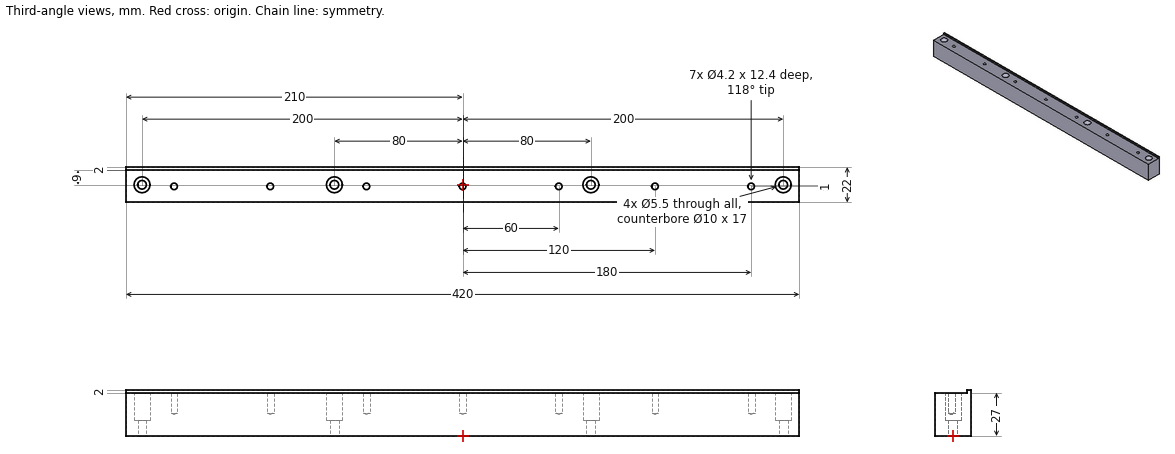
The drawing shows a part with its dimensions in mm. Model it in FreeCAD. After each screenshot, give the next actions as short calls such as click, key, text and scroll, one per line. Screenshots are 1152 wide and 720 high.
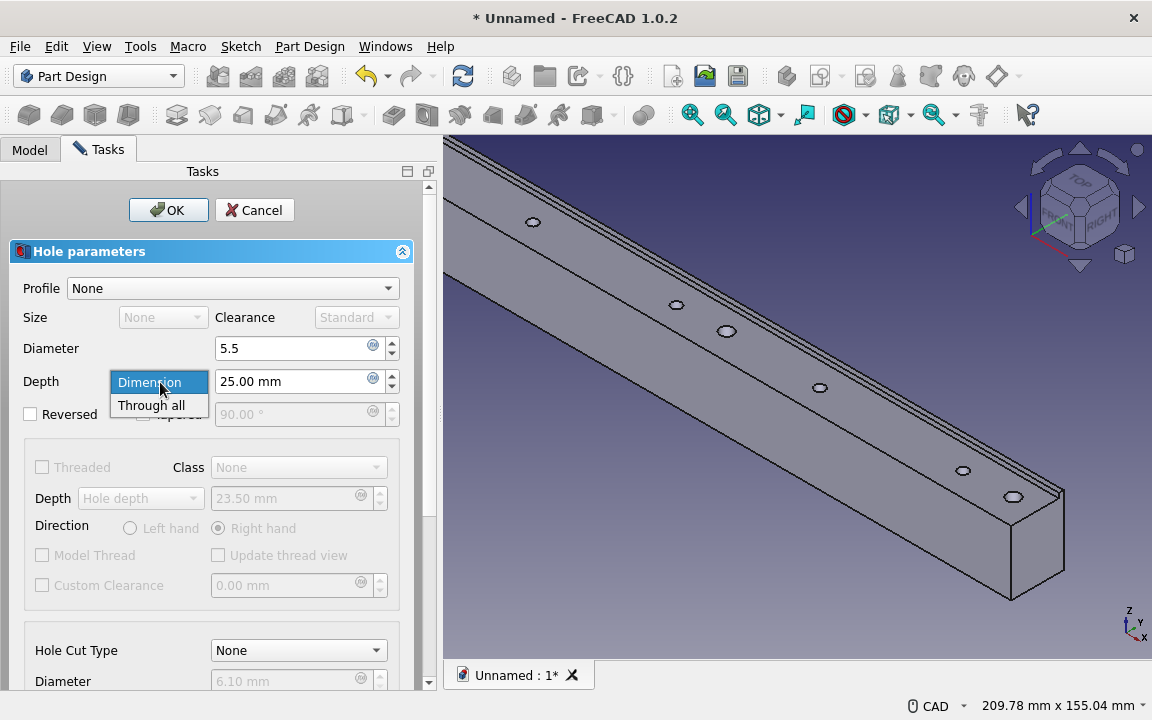
click(158, 406)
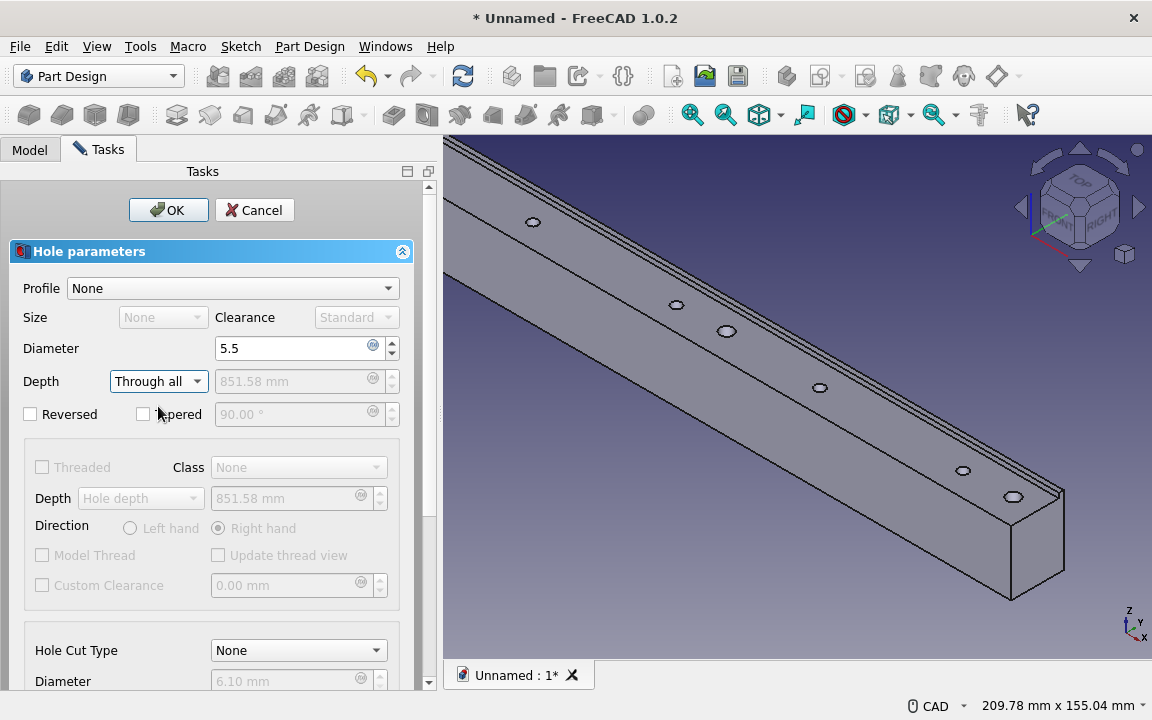
click(300, 650)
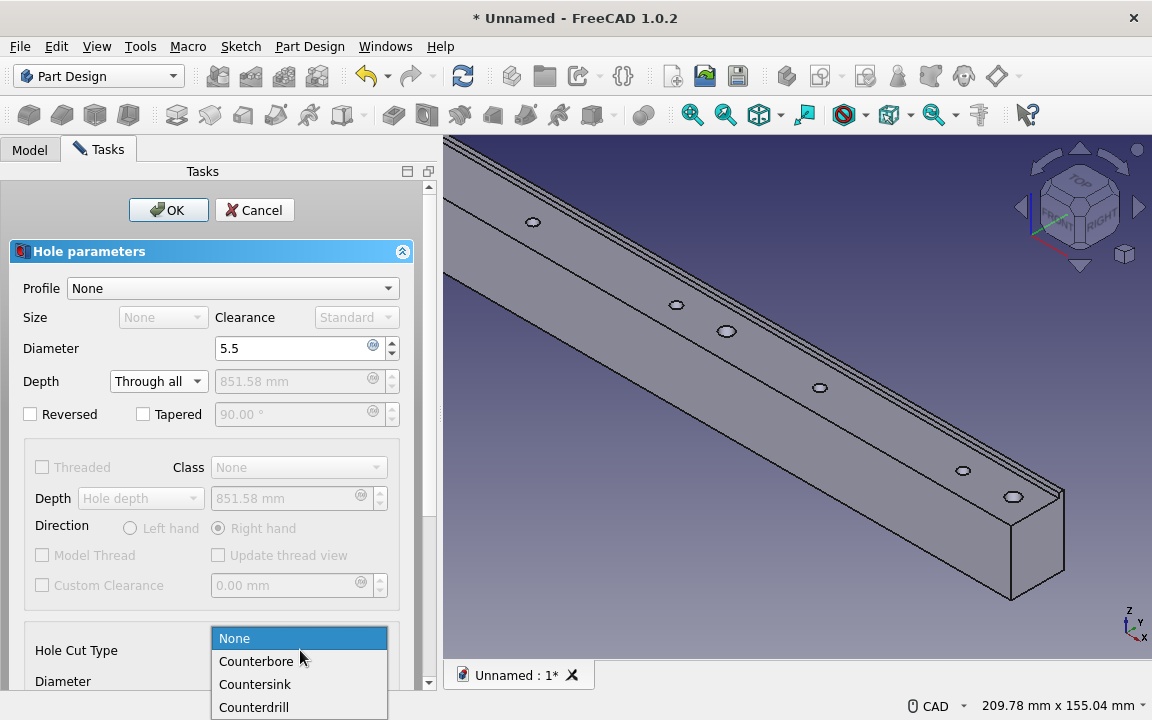
click(298, 662)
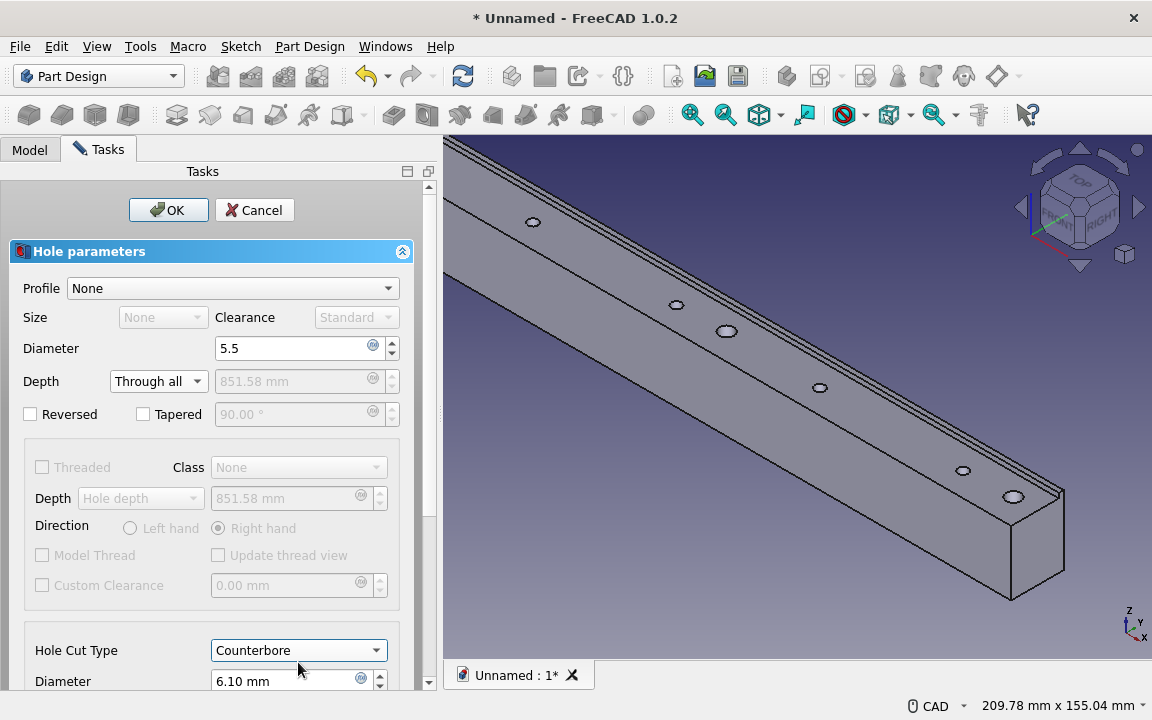
scroll(429, 436, down, 2)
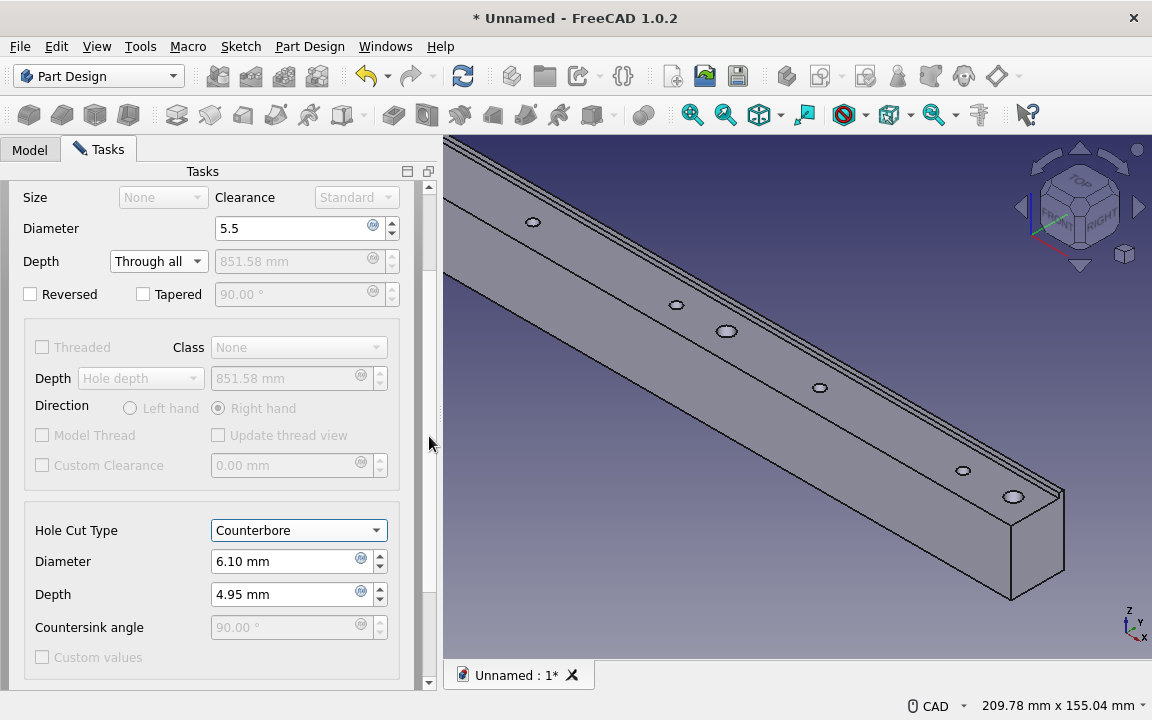
triple_click(292, 562)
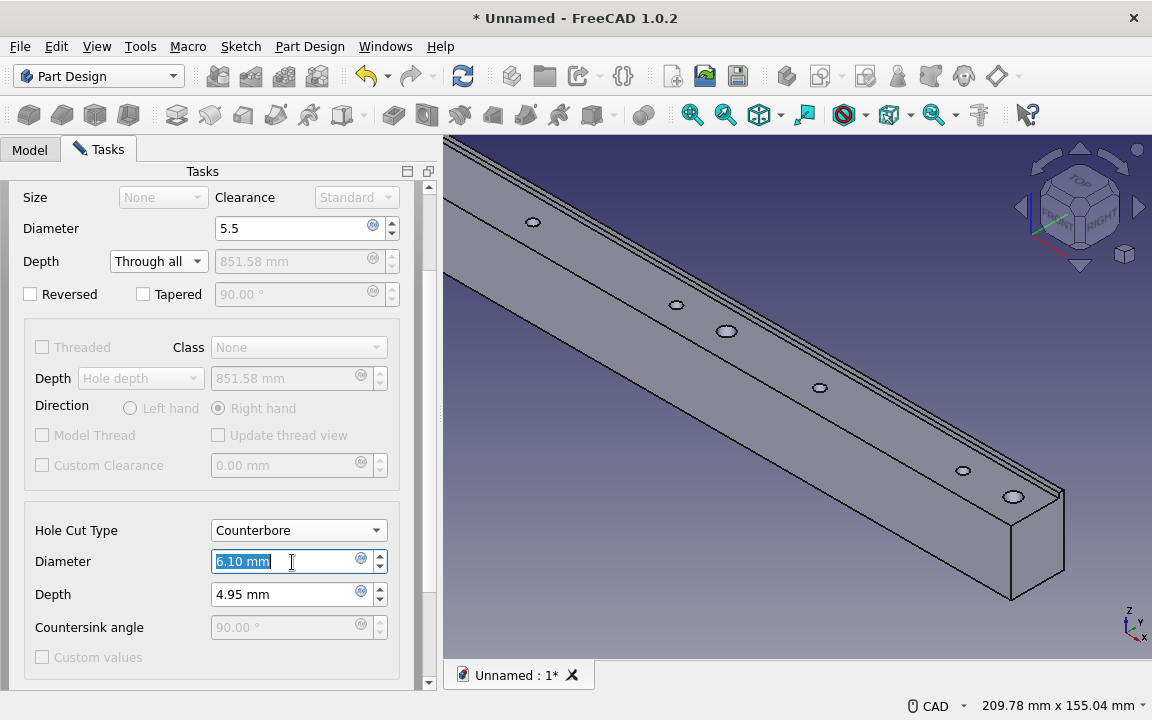
text(10)
key(Tab)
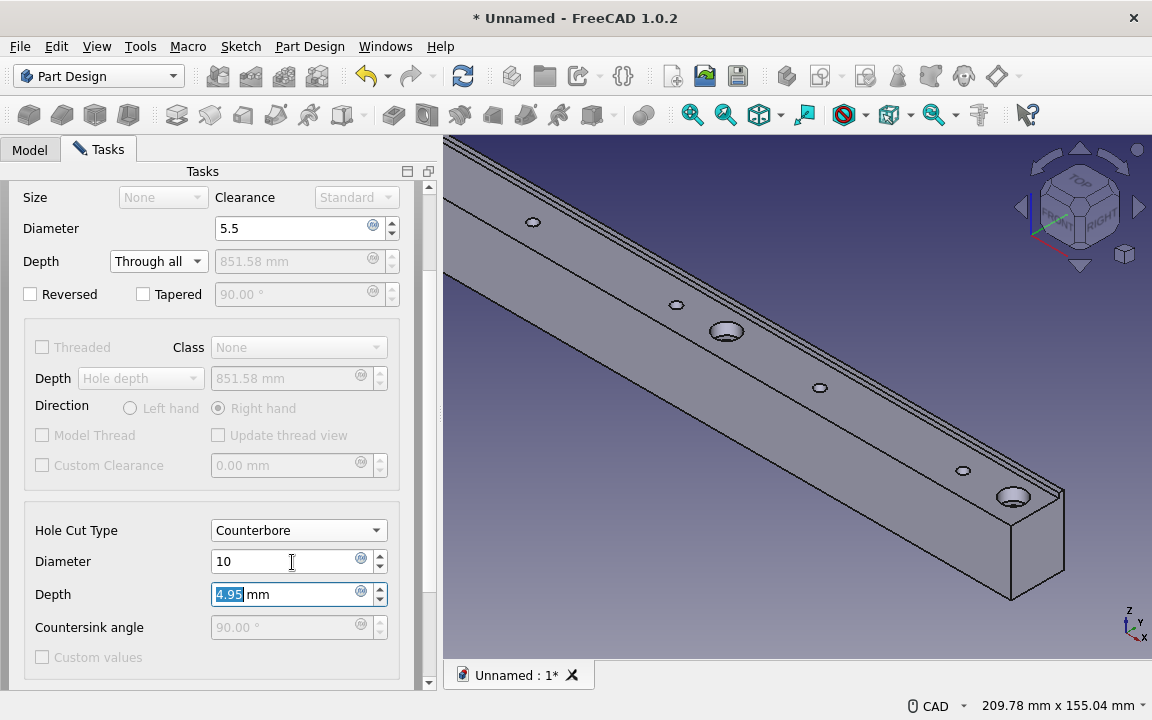
text(17)
key(Tab)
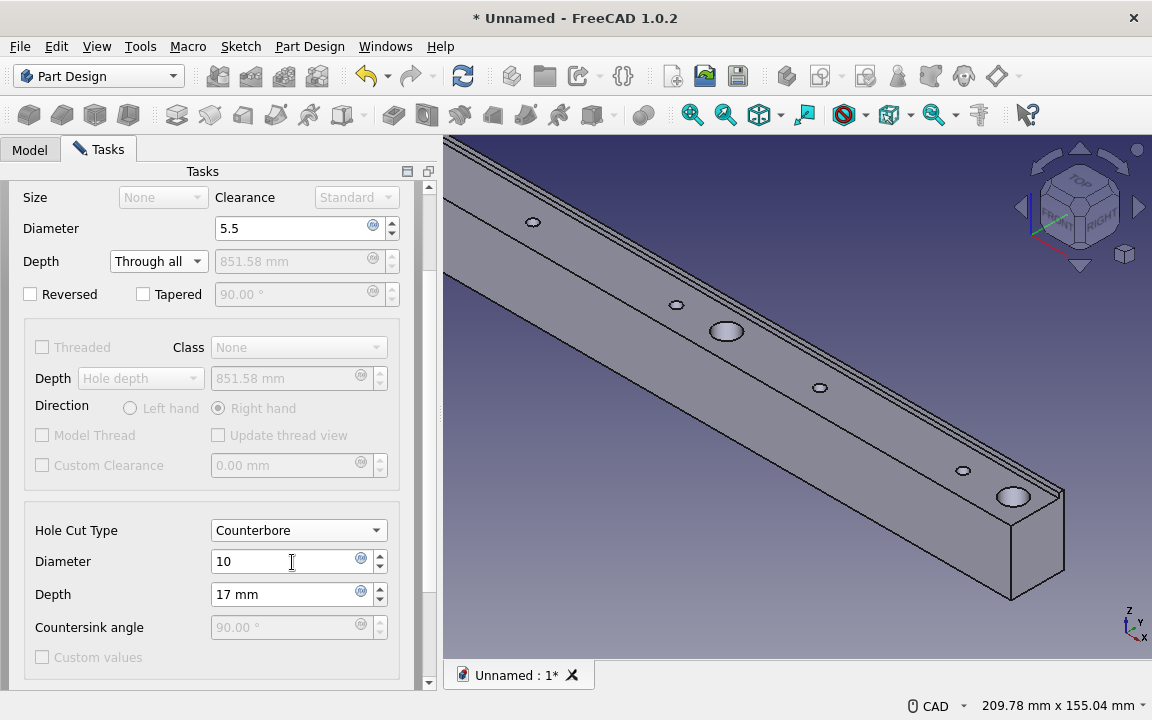
scroll(429, 436, up, 3)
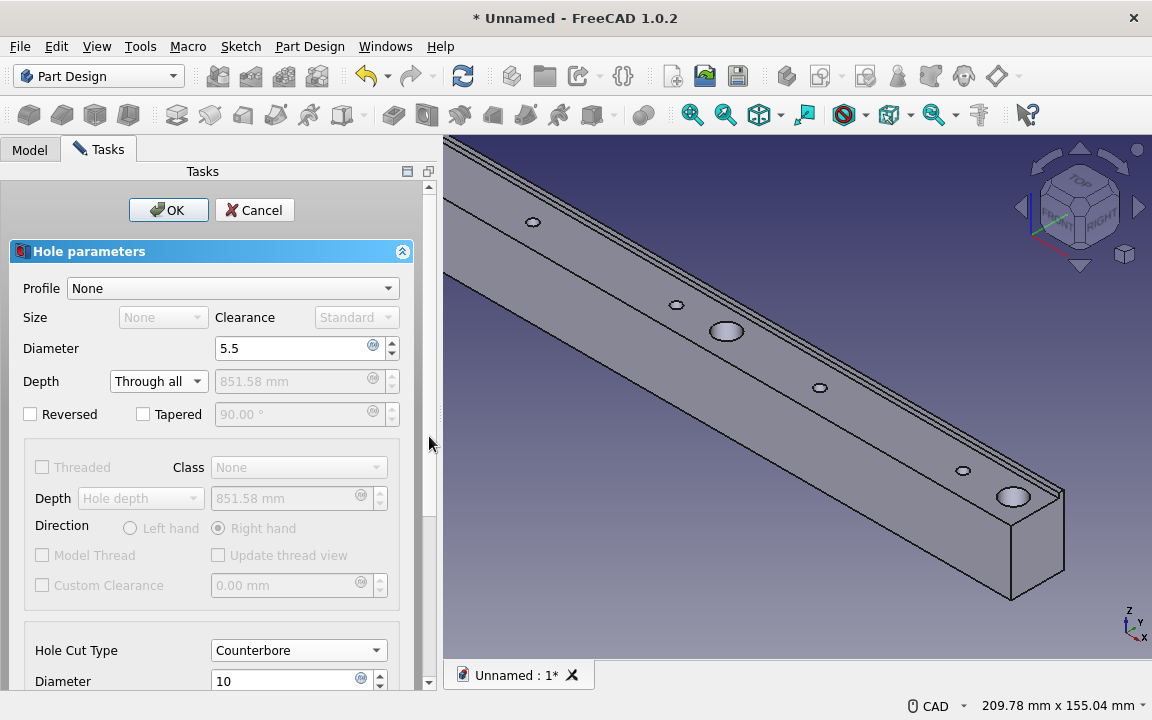
click(169, 210)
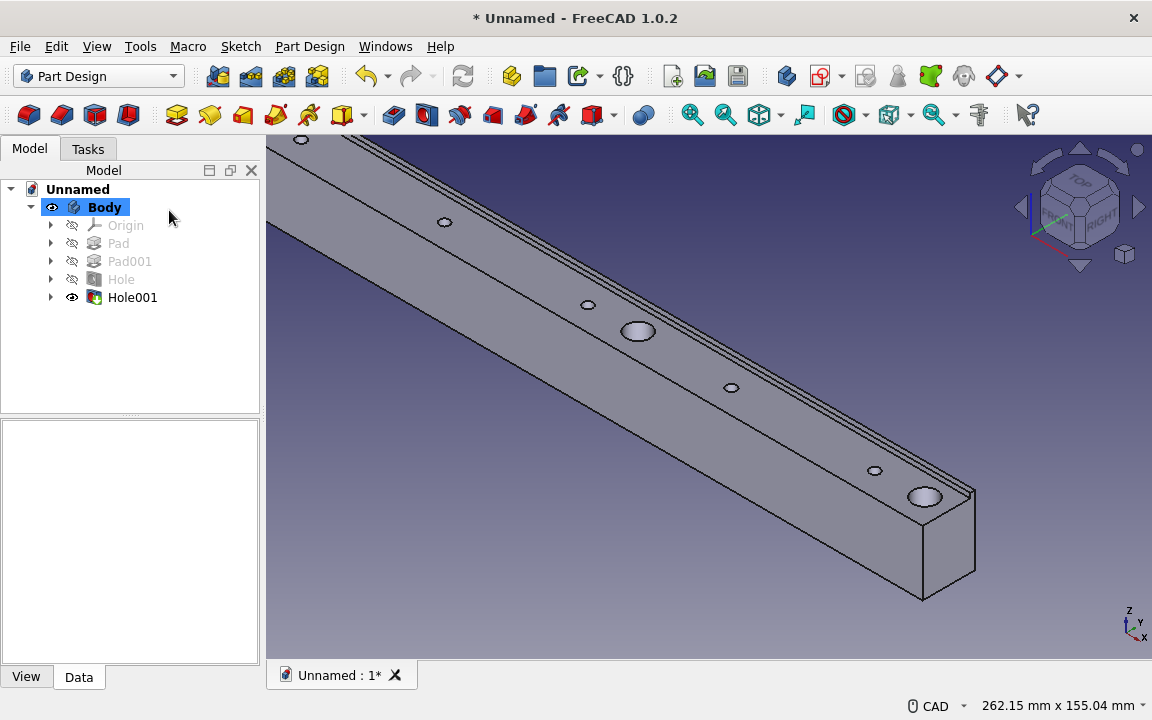
click(693, 116)